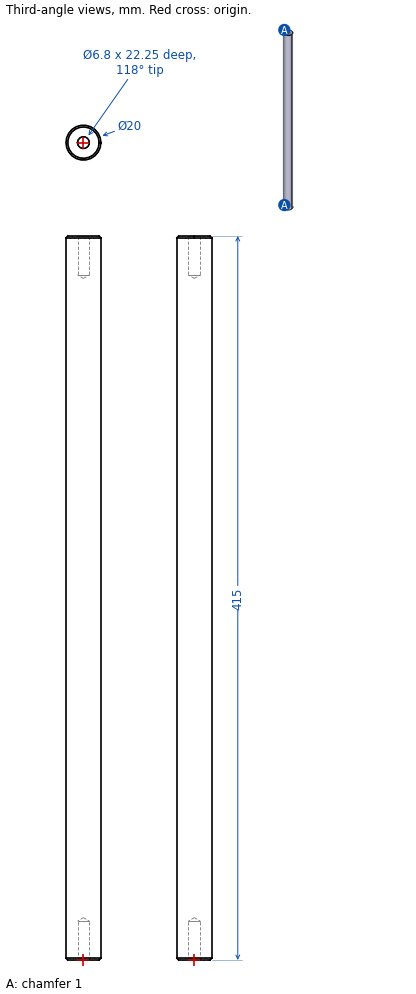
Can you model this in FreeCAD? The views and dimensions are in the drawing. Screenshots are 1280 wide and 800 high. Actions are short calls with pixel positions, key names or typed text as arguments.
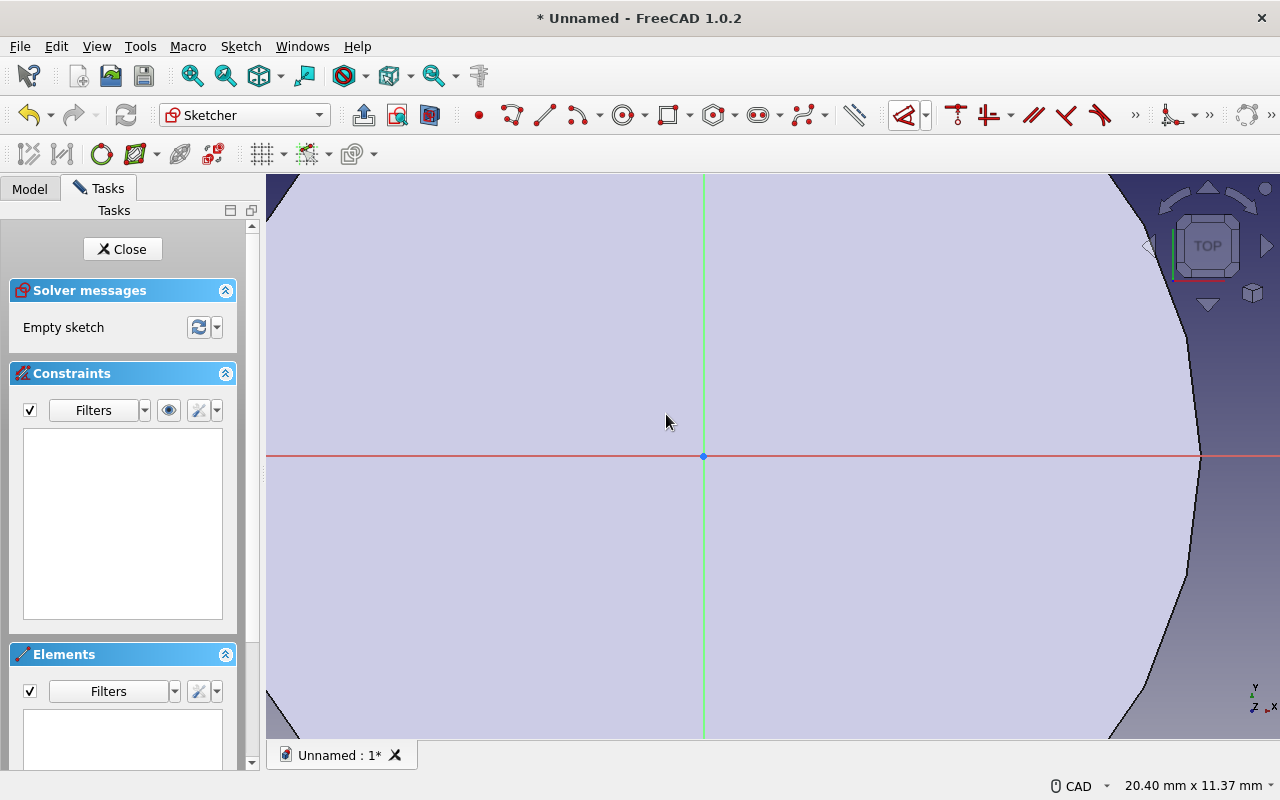
click(622, 116)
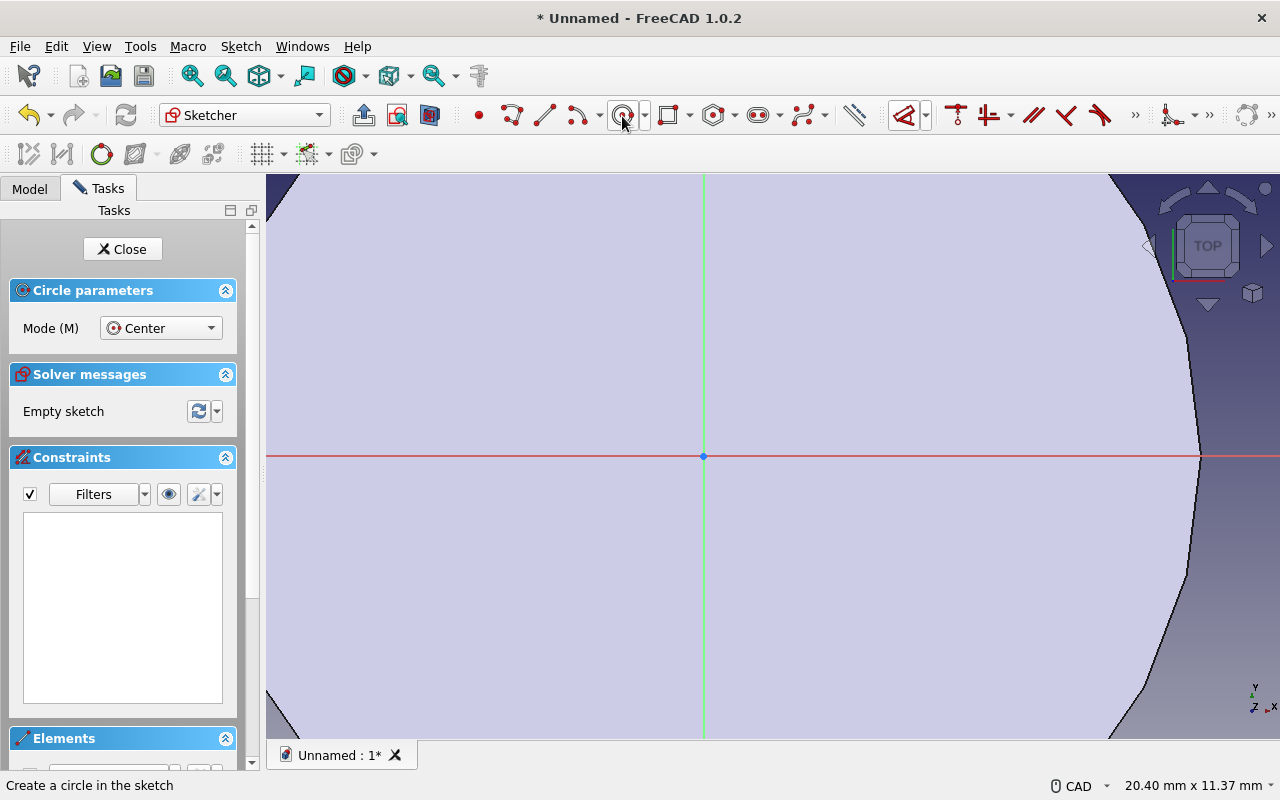
click(704, 456)
click(824, 337)
key(Escape)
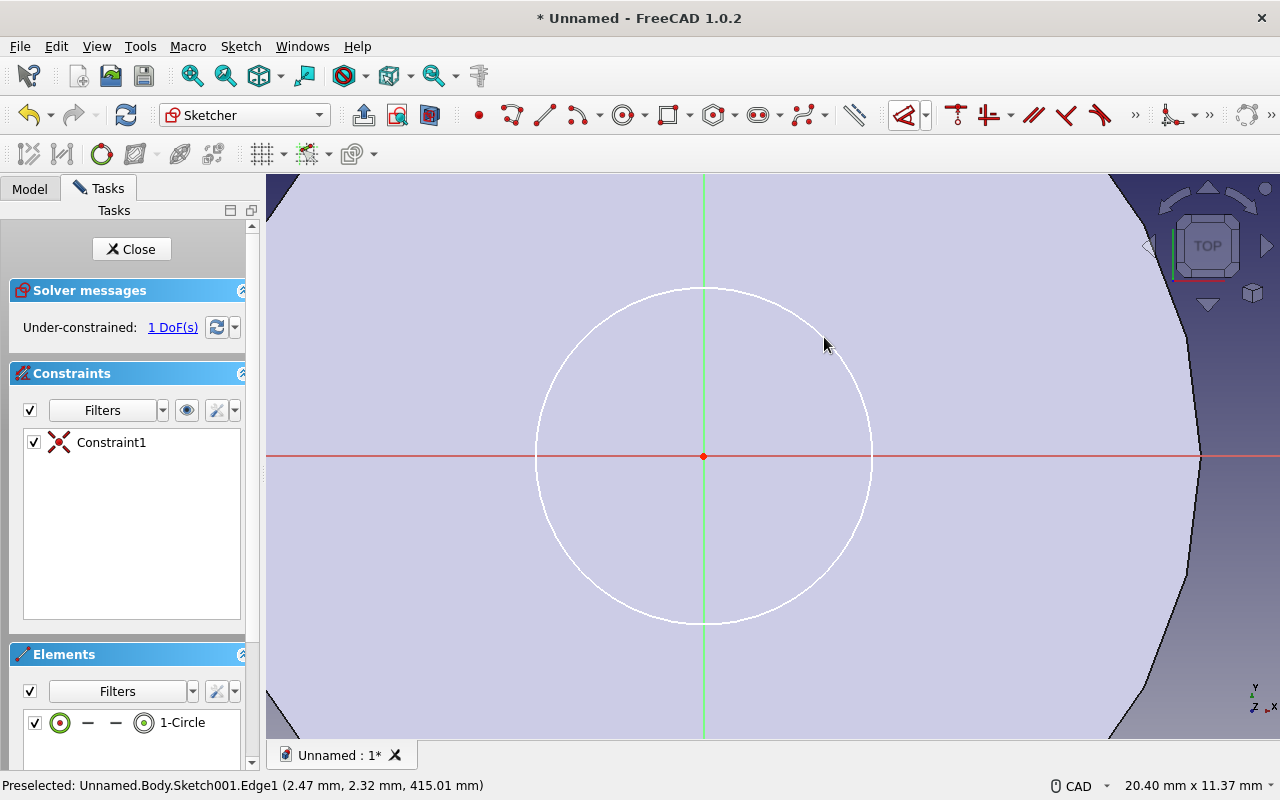
click(823, 337)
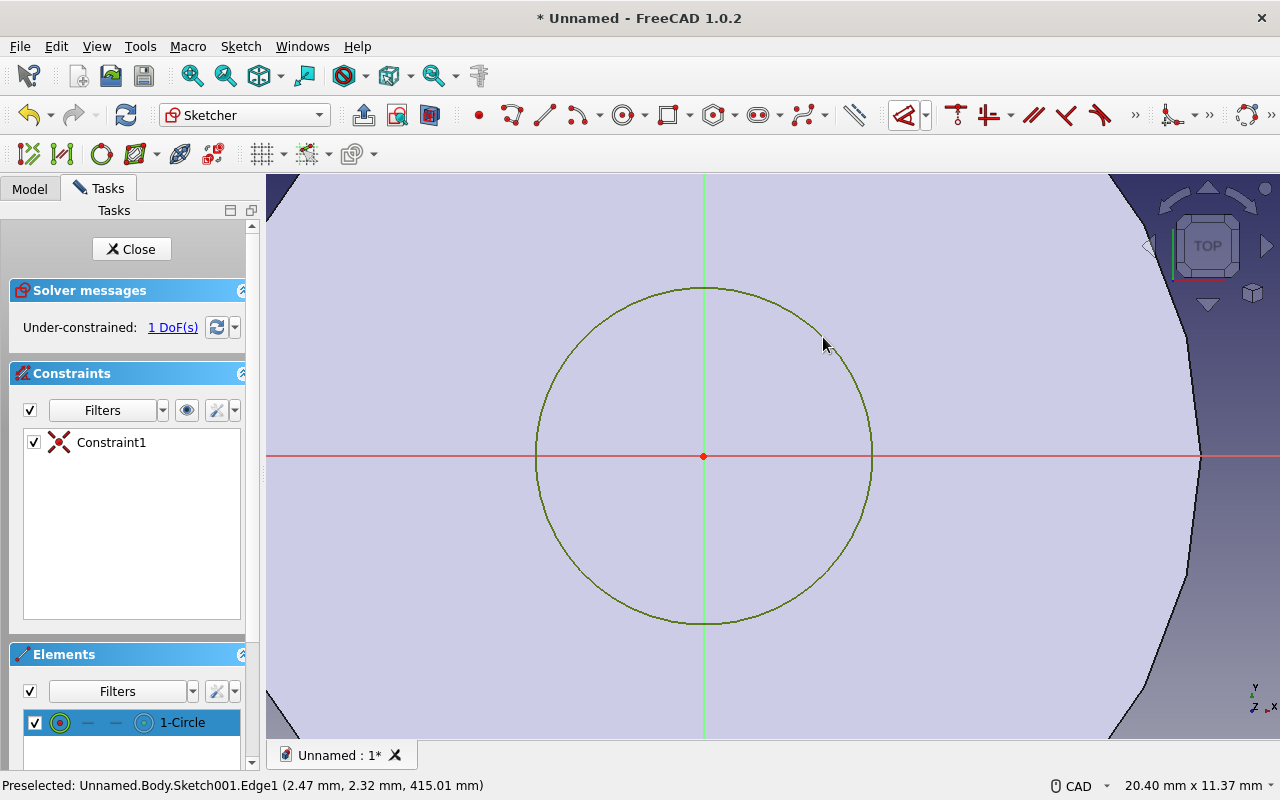
key(k)
key(o)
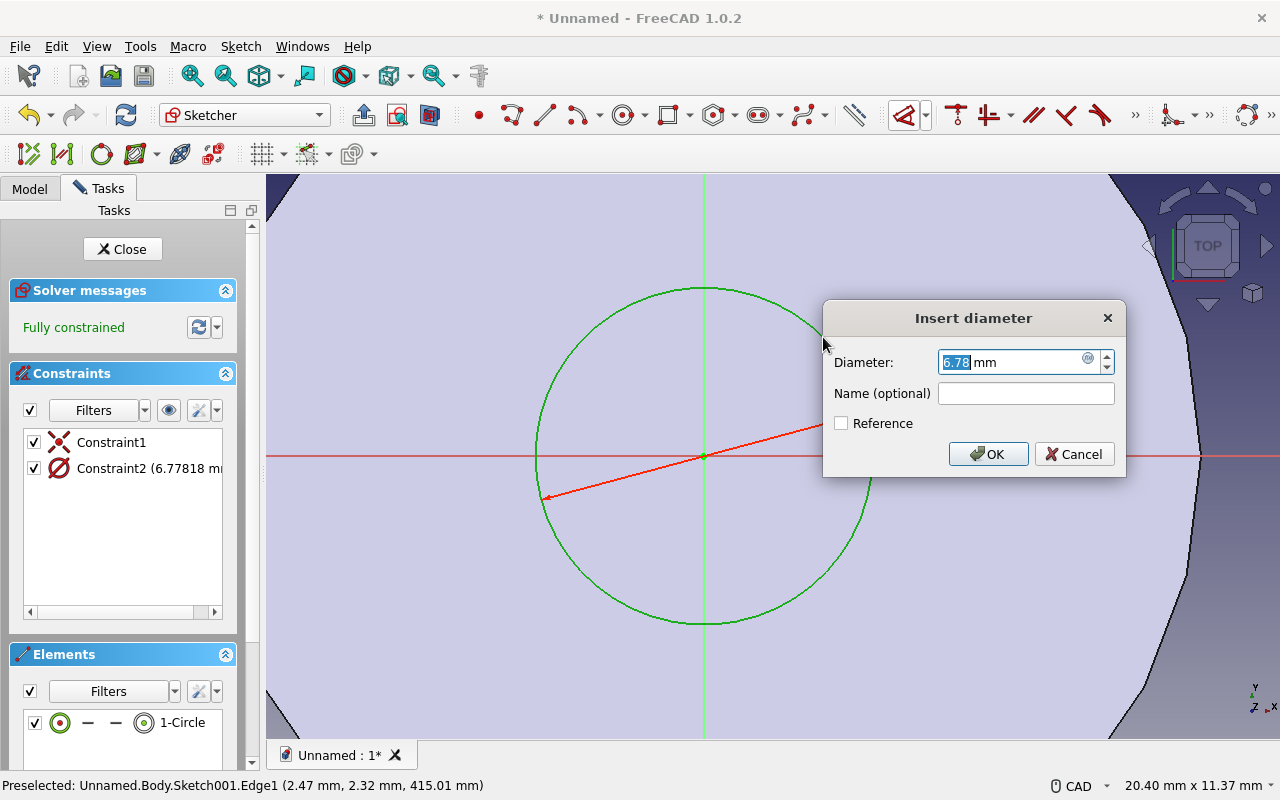
text(6.8)
key(Return)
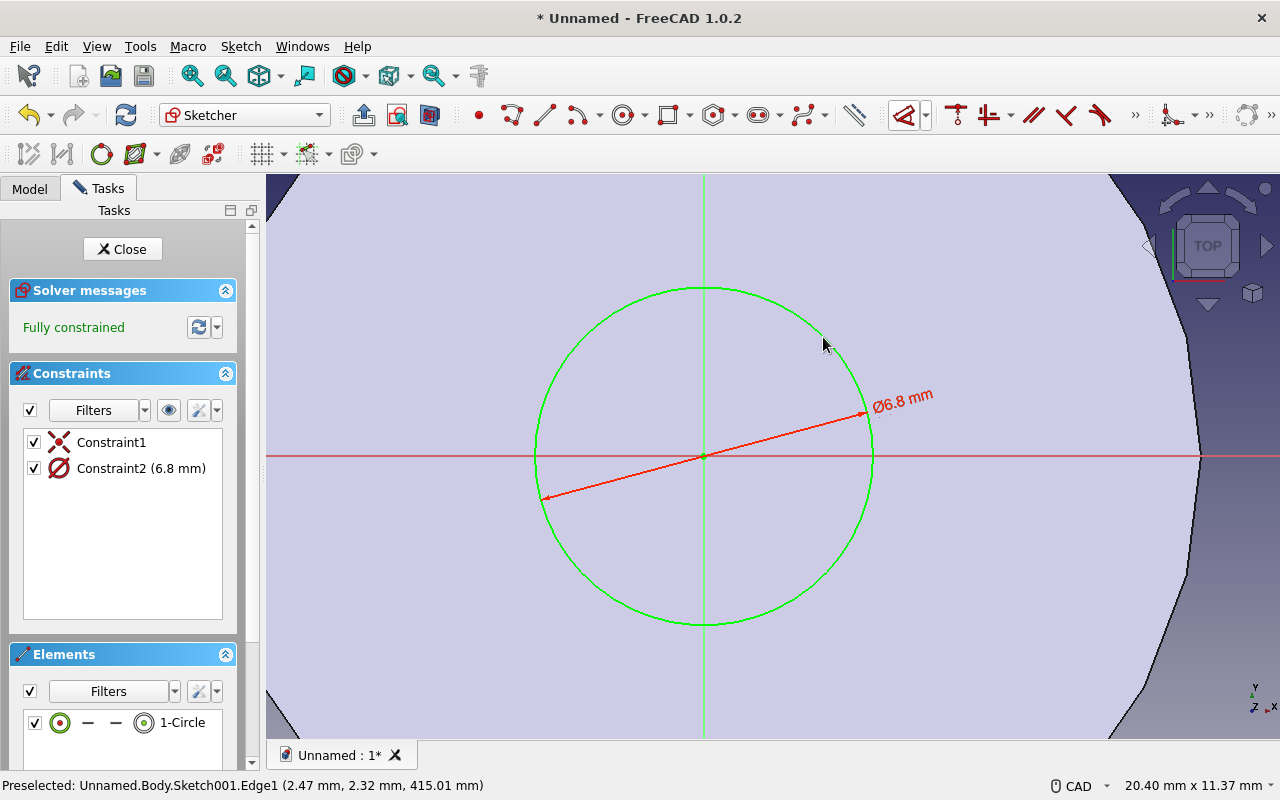
click(123, 249)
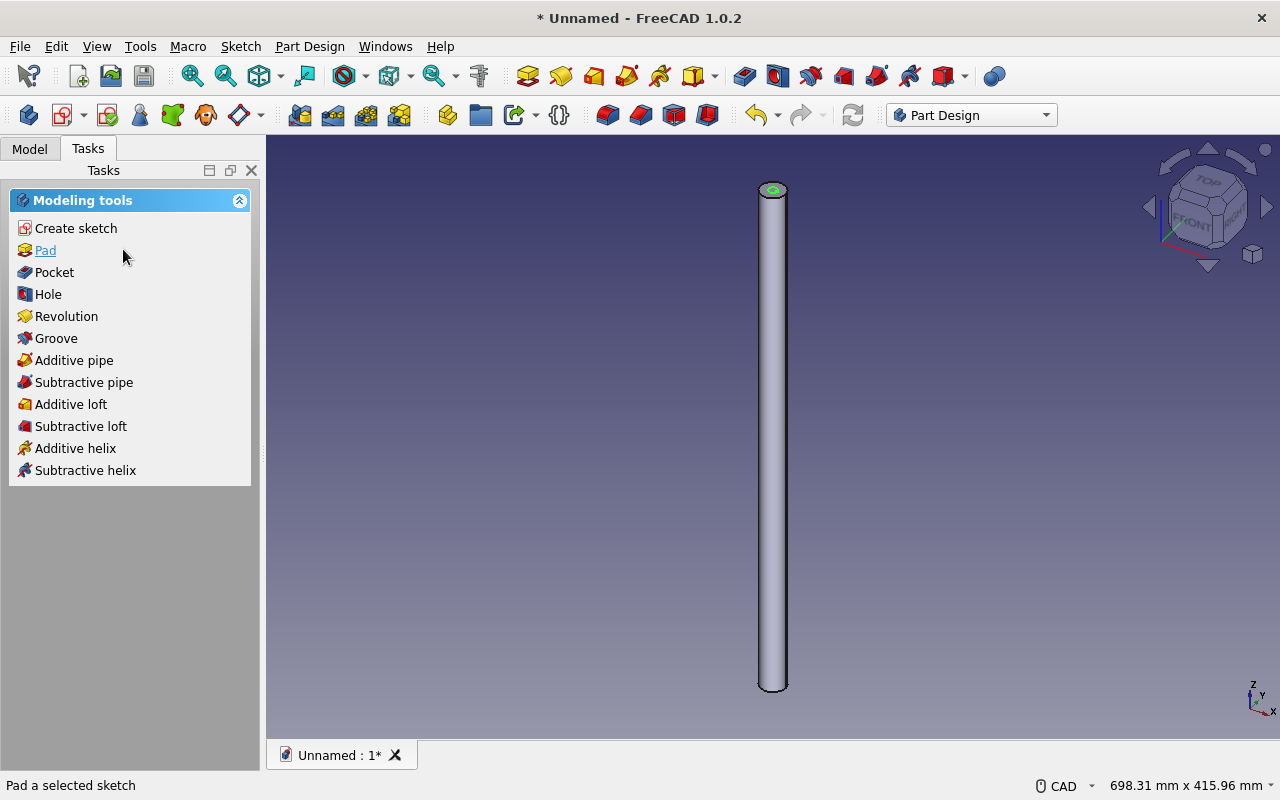
click(778, 76)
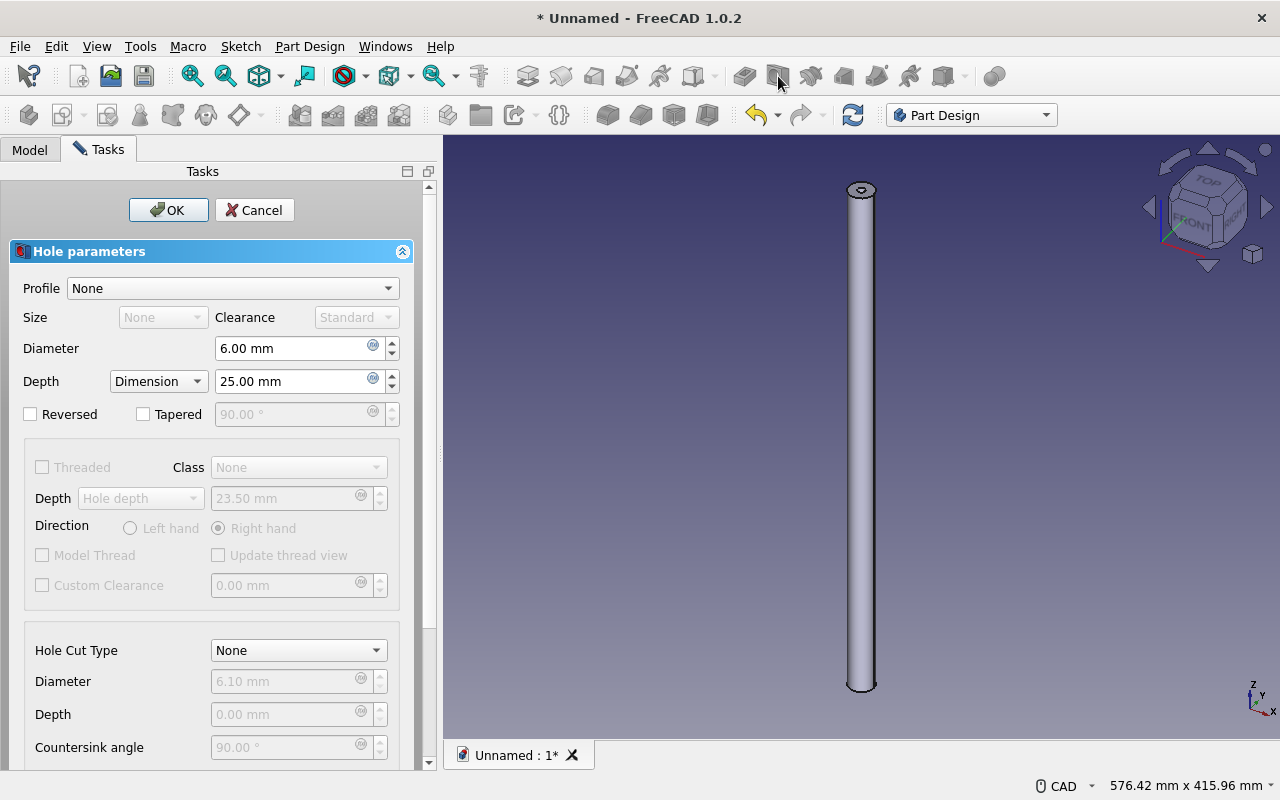
triple_click(300, 348)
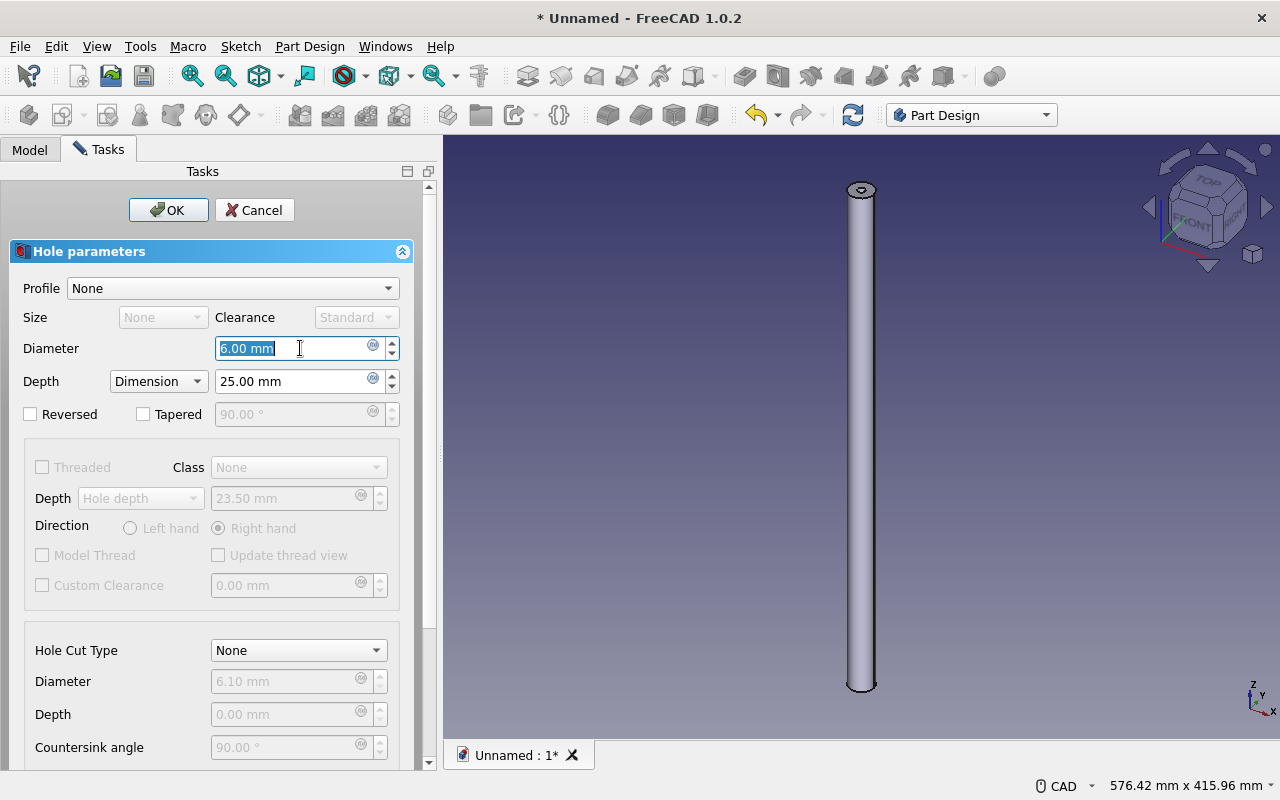
text(6.8)
key(Tab)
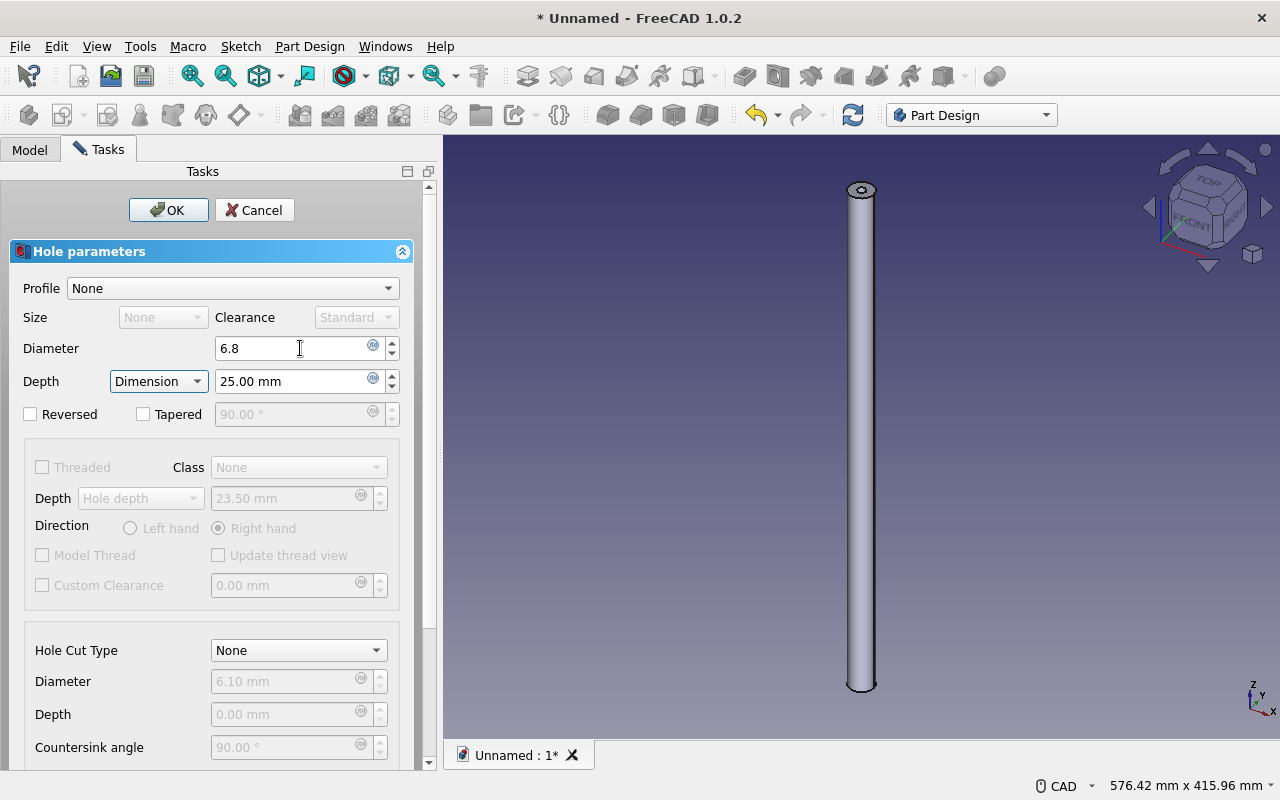
triple_click(300, 382)